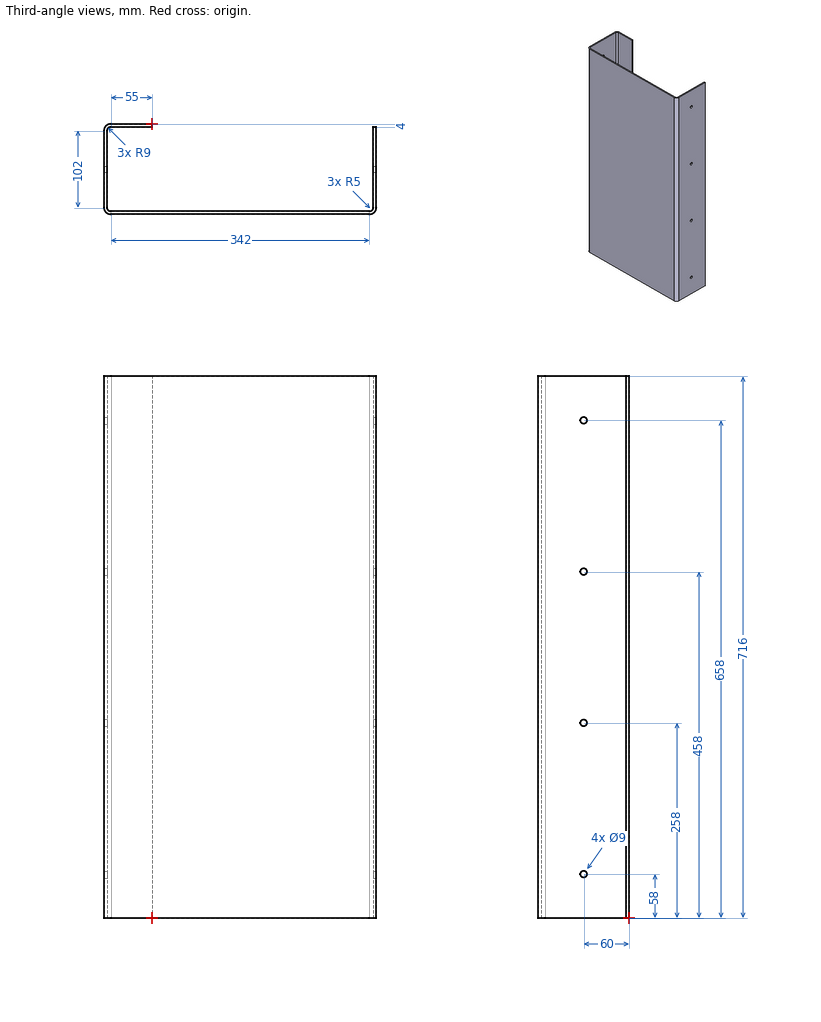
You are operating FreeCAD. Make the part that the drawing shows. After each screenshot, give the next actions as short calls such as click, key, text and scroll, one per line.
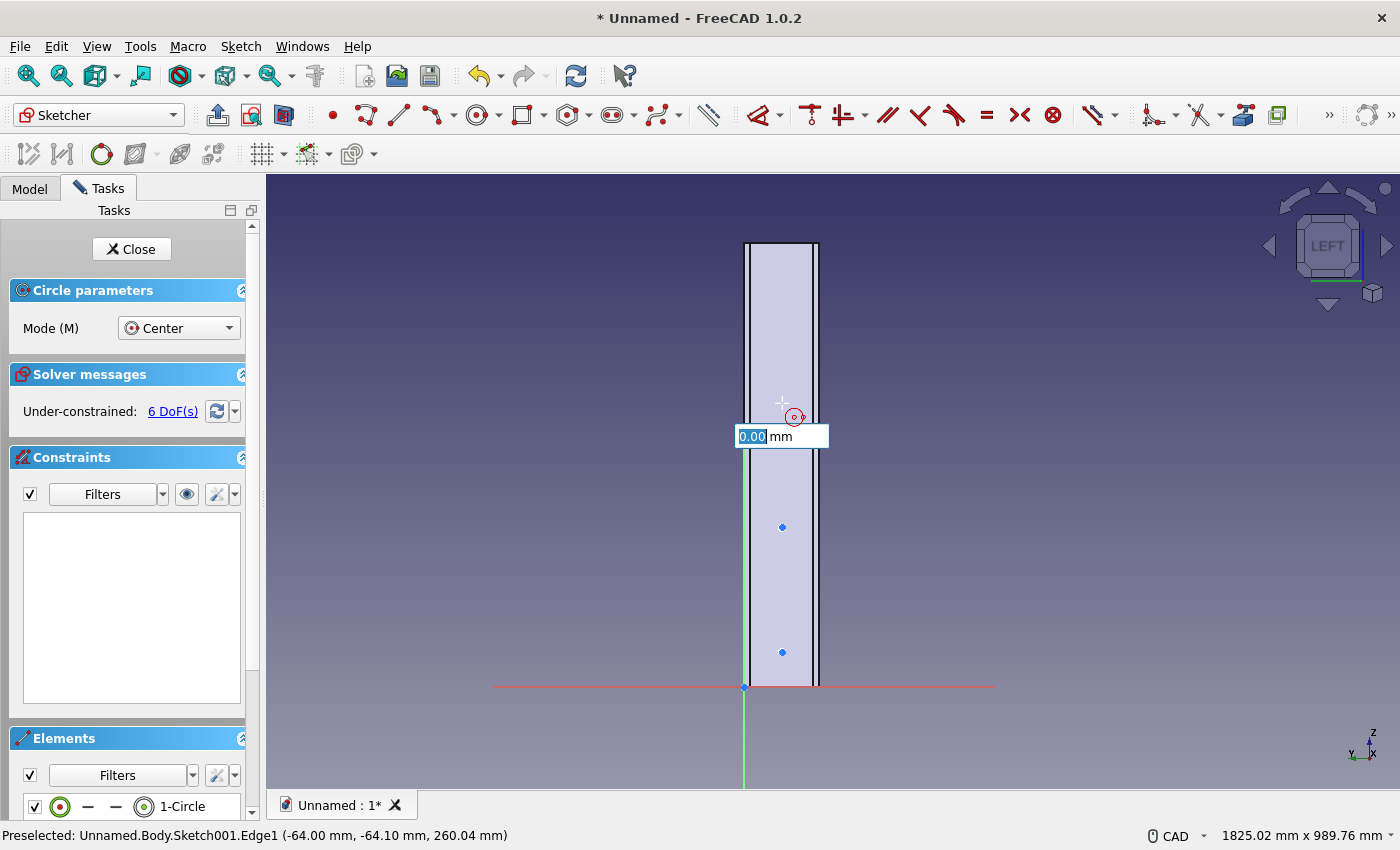
scroll(784, 401, up, 9)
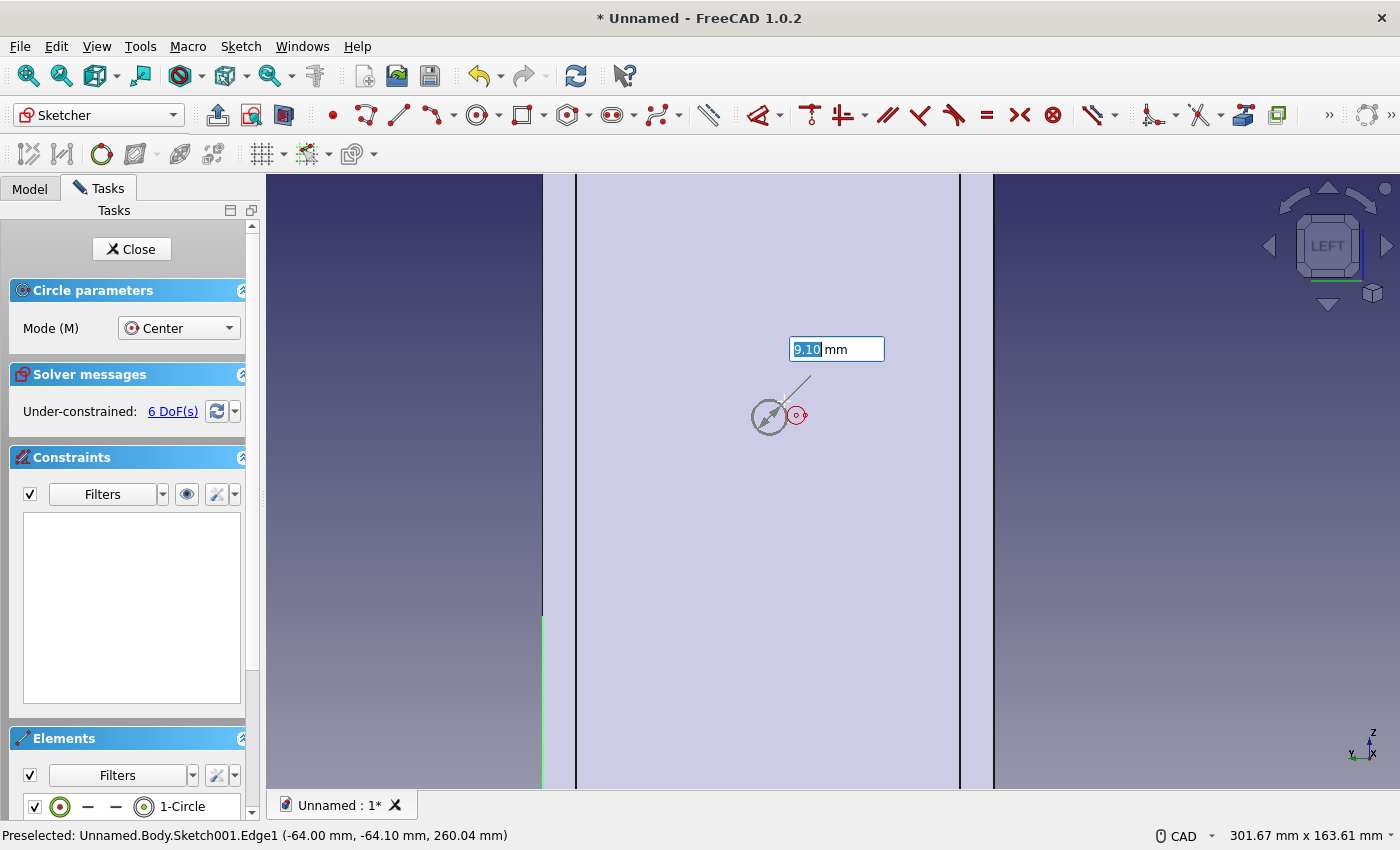
click(780, 398)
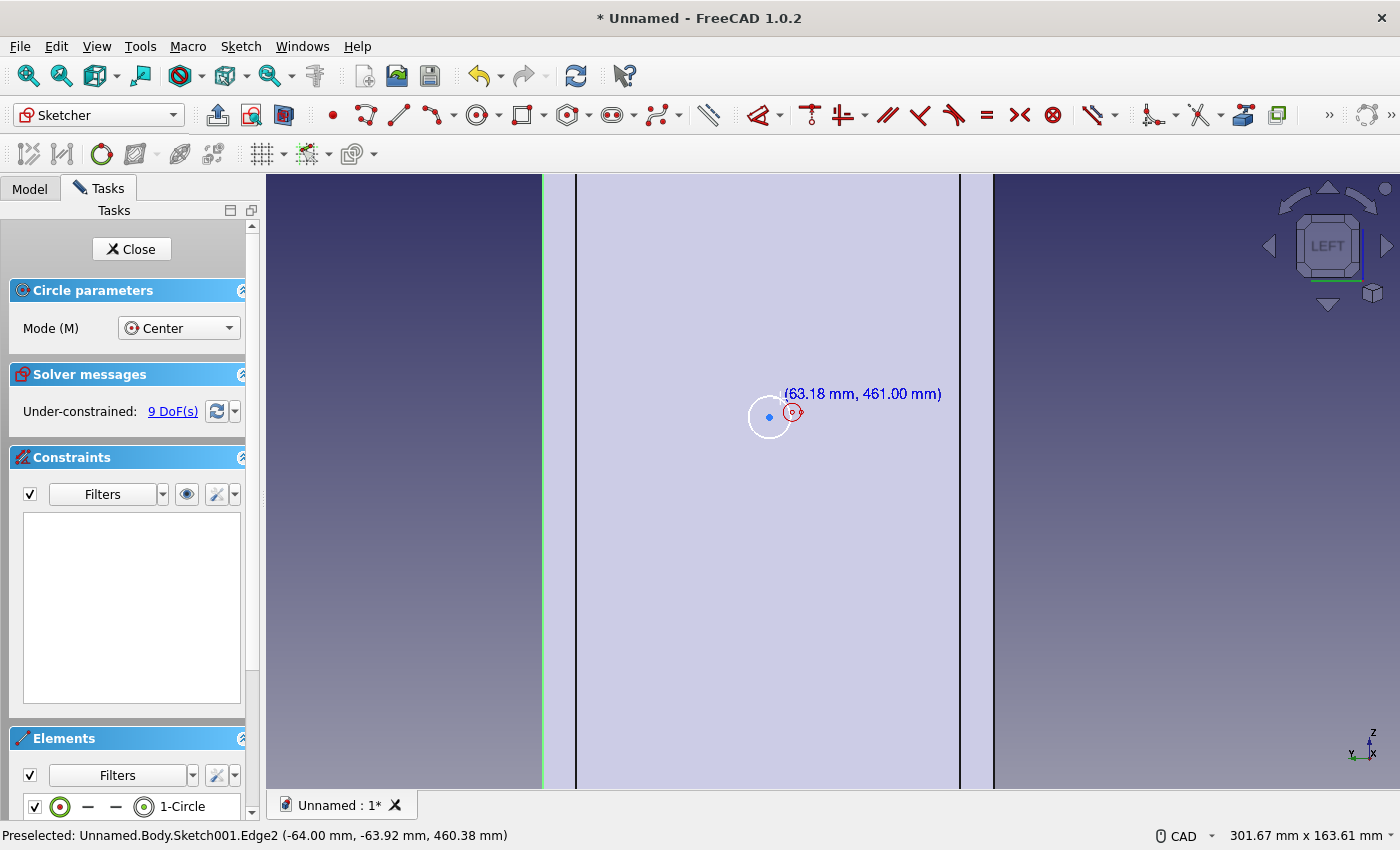
scroll(784, 401, down, 9)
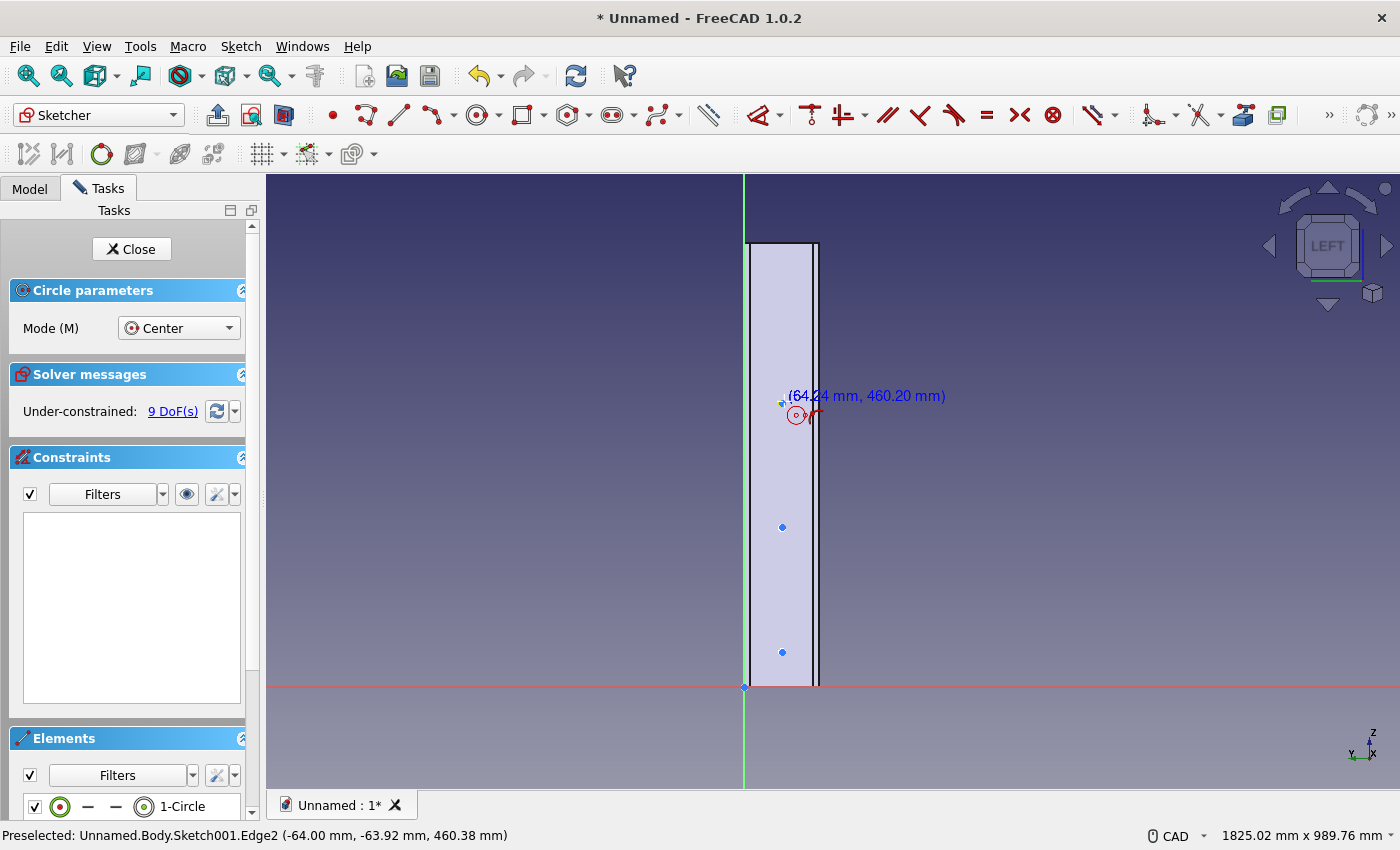
scroll(782, 279, up, 11)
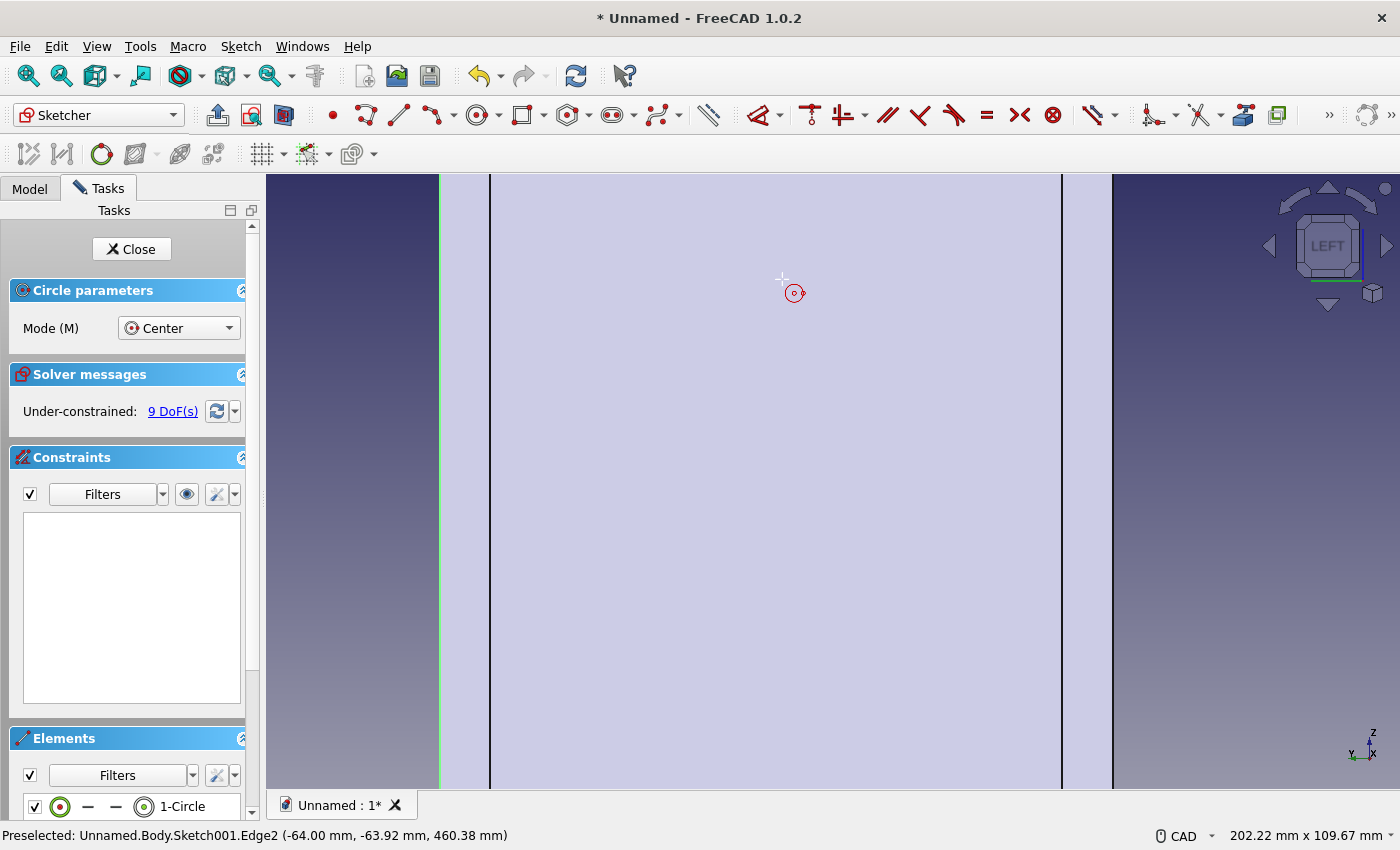
scroll(782, 279, down, 11)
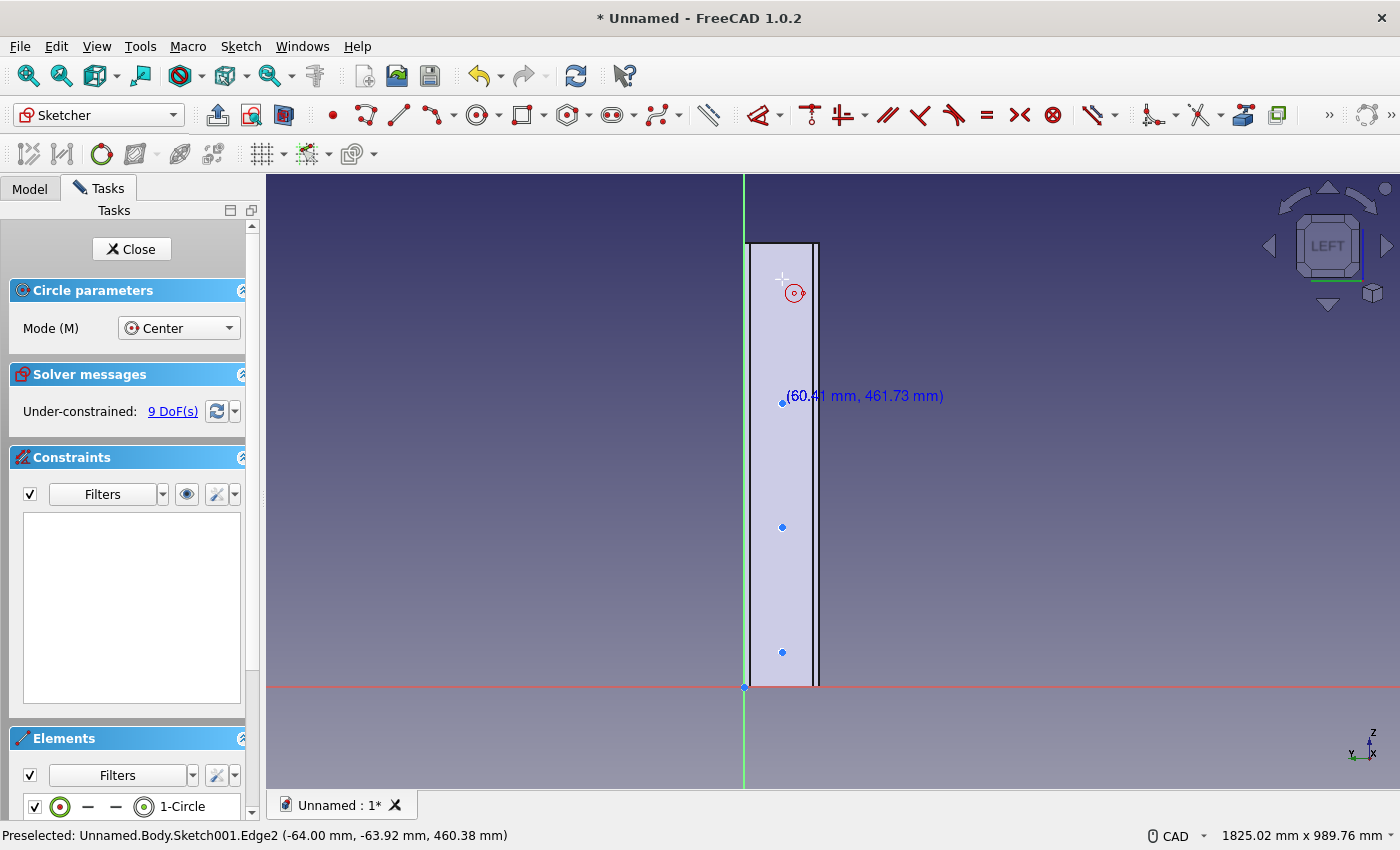
click(782, 279)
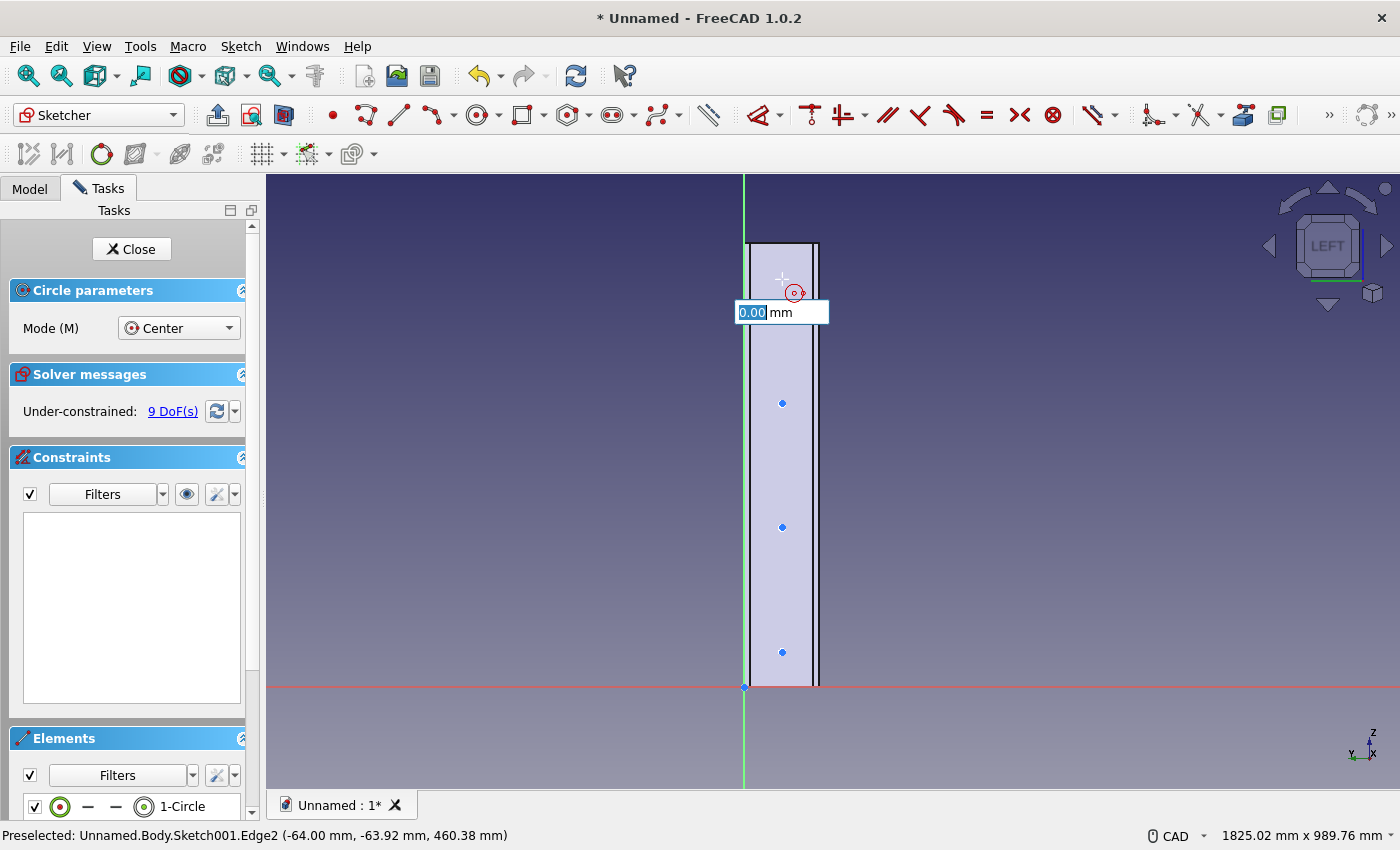
scroll(784, 277, up, 9)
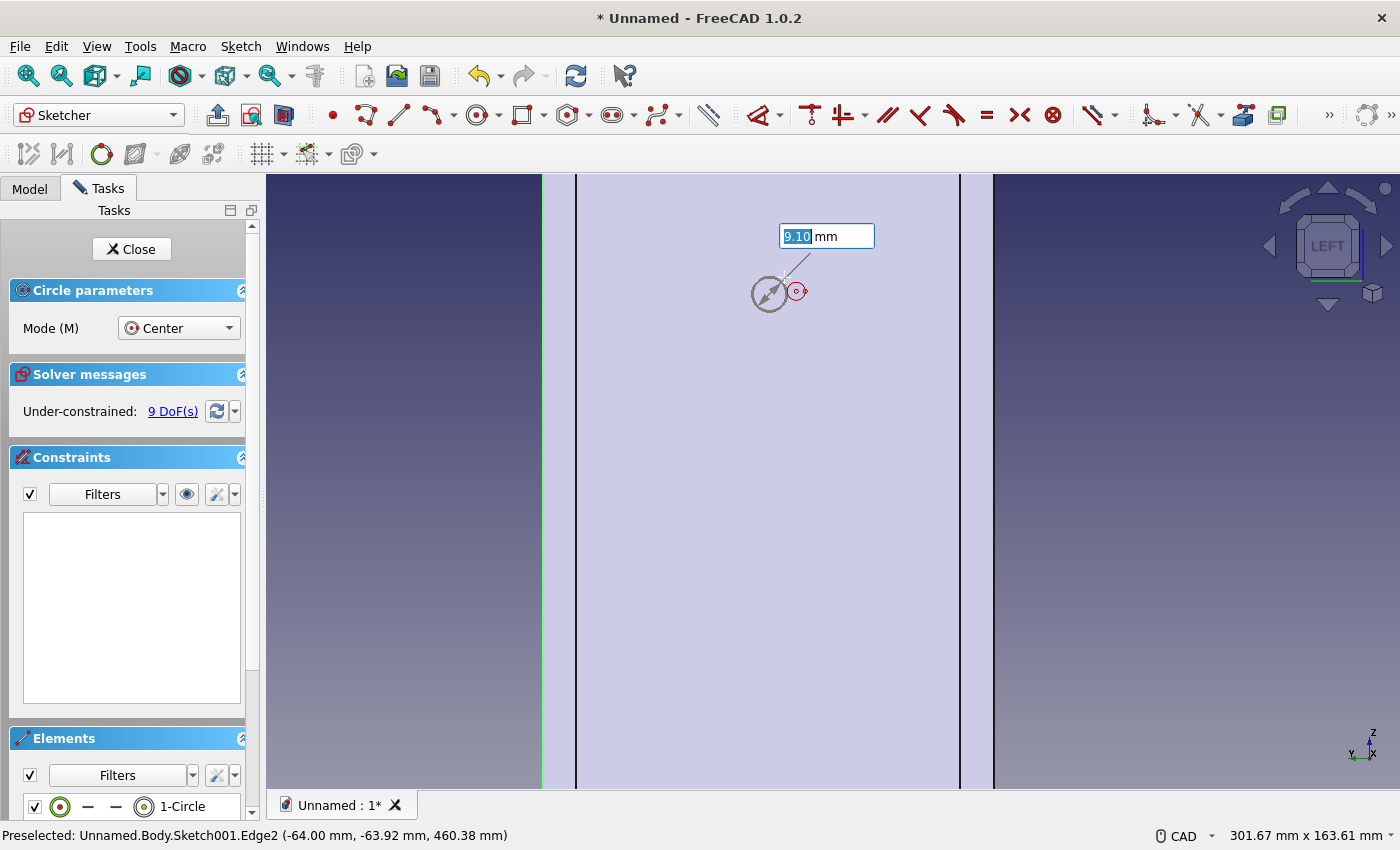
click(780, 274)
key(Escape)